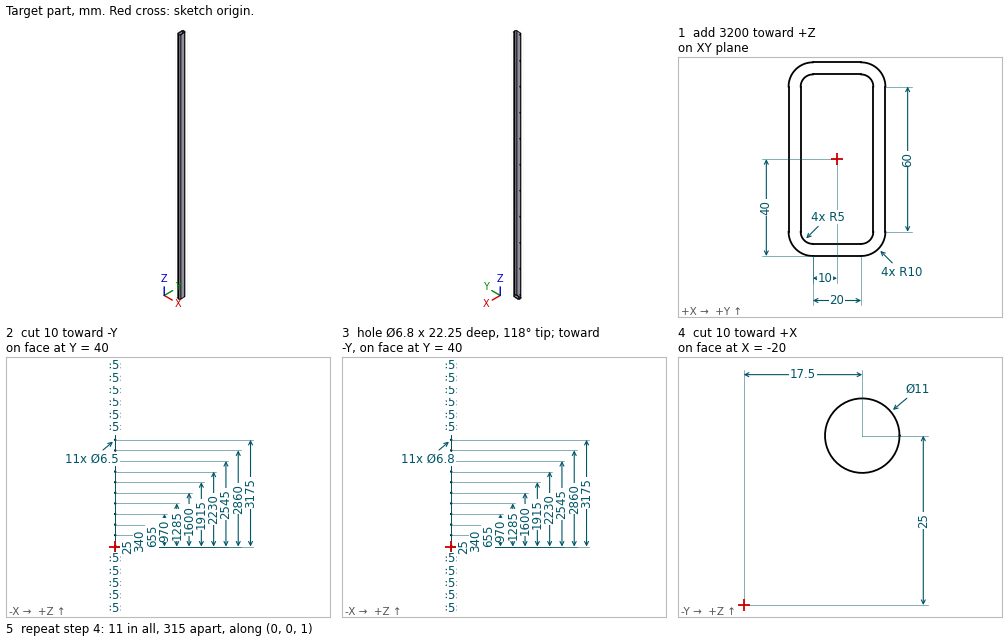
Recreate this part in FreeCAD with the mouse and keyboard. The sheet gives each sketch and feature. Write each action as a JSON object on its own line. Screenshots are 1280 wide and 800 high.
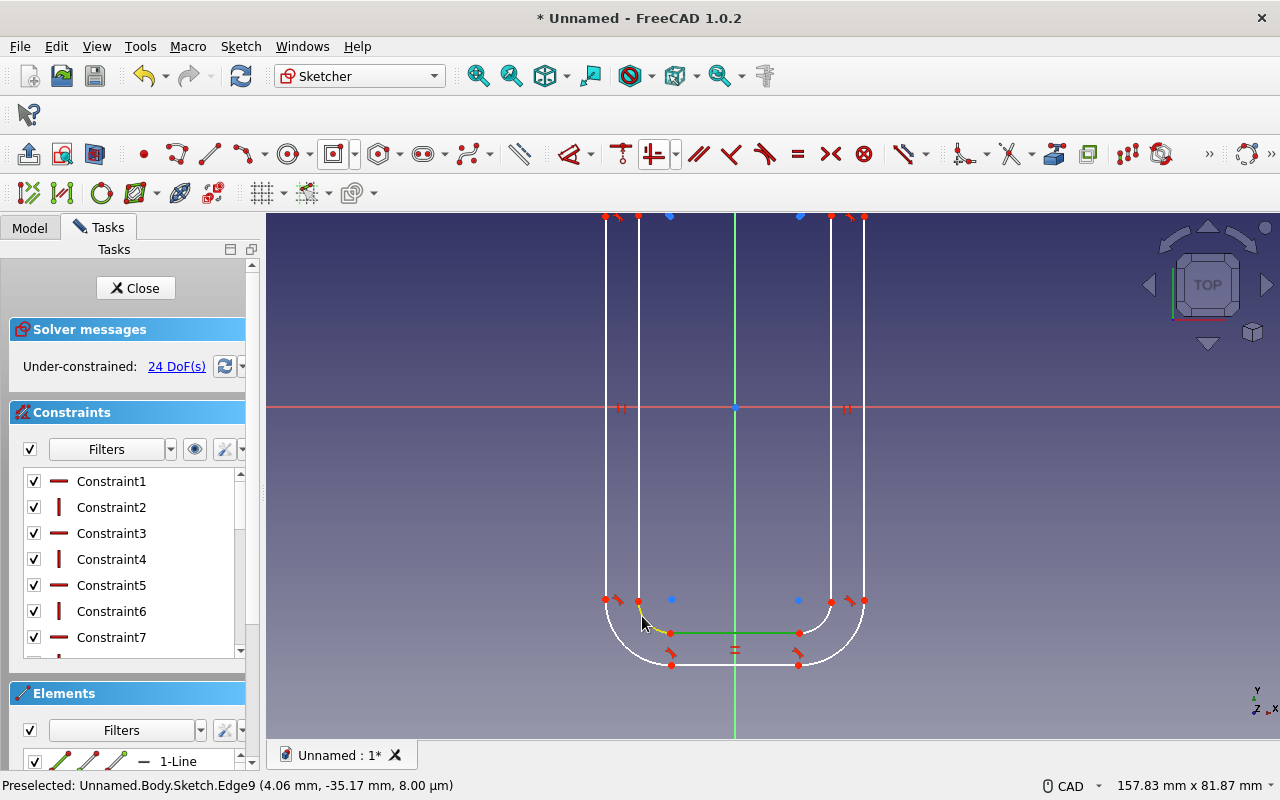
{"action": "left_click", "coordinate": [643, 616]}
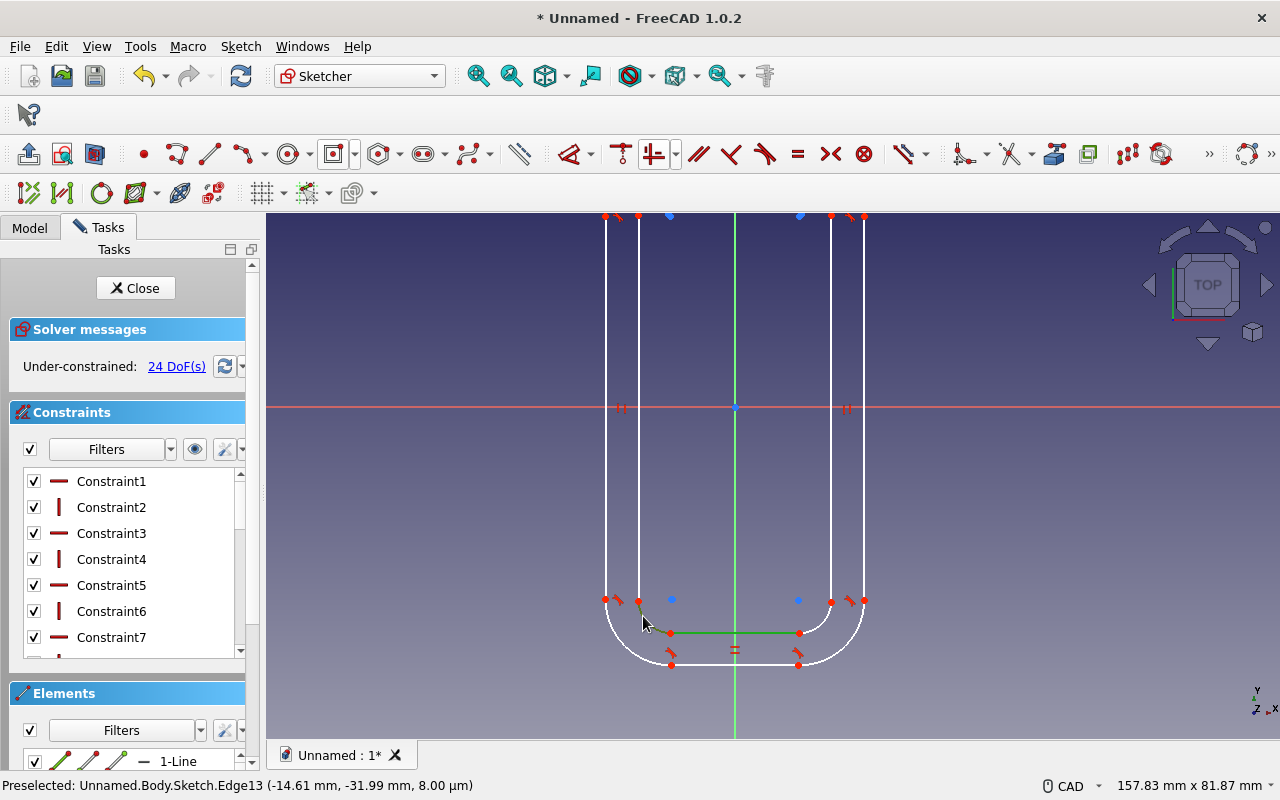
{"action": "left_click", "coordinate": [765, 154]}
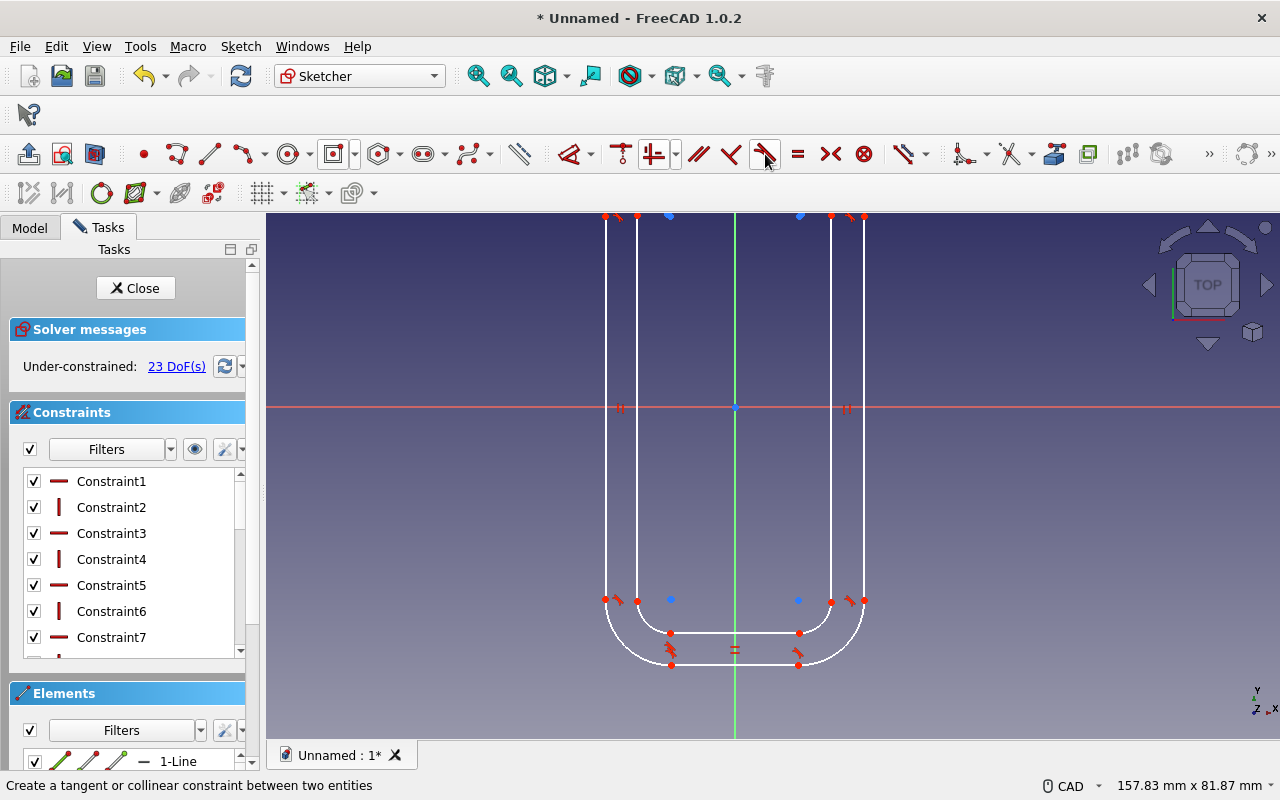
{"action": "left_click", "coordinate": [761, 633]}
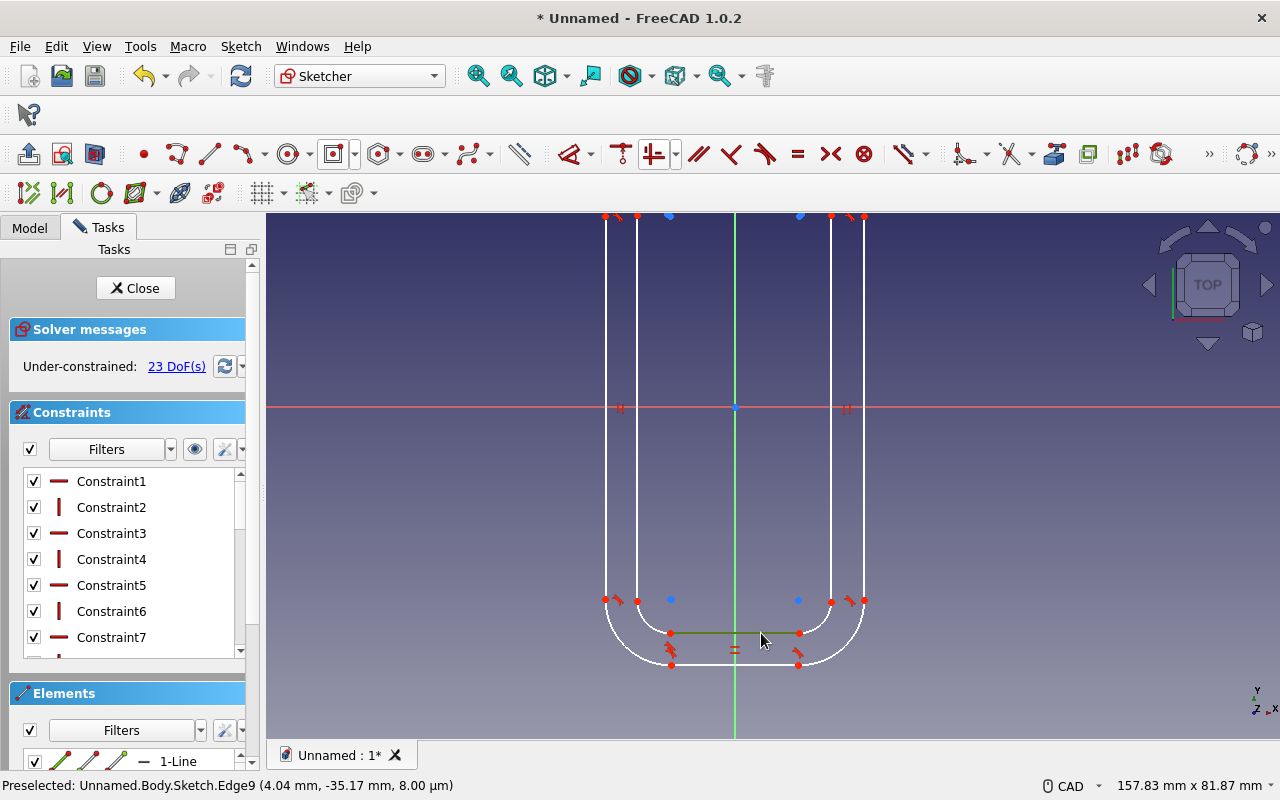
{"action": "left_click", "coordinate": [814, 630]}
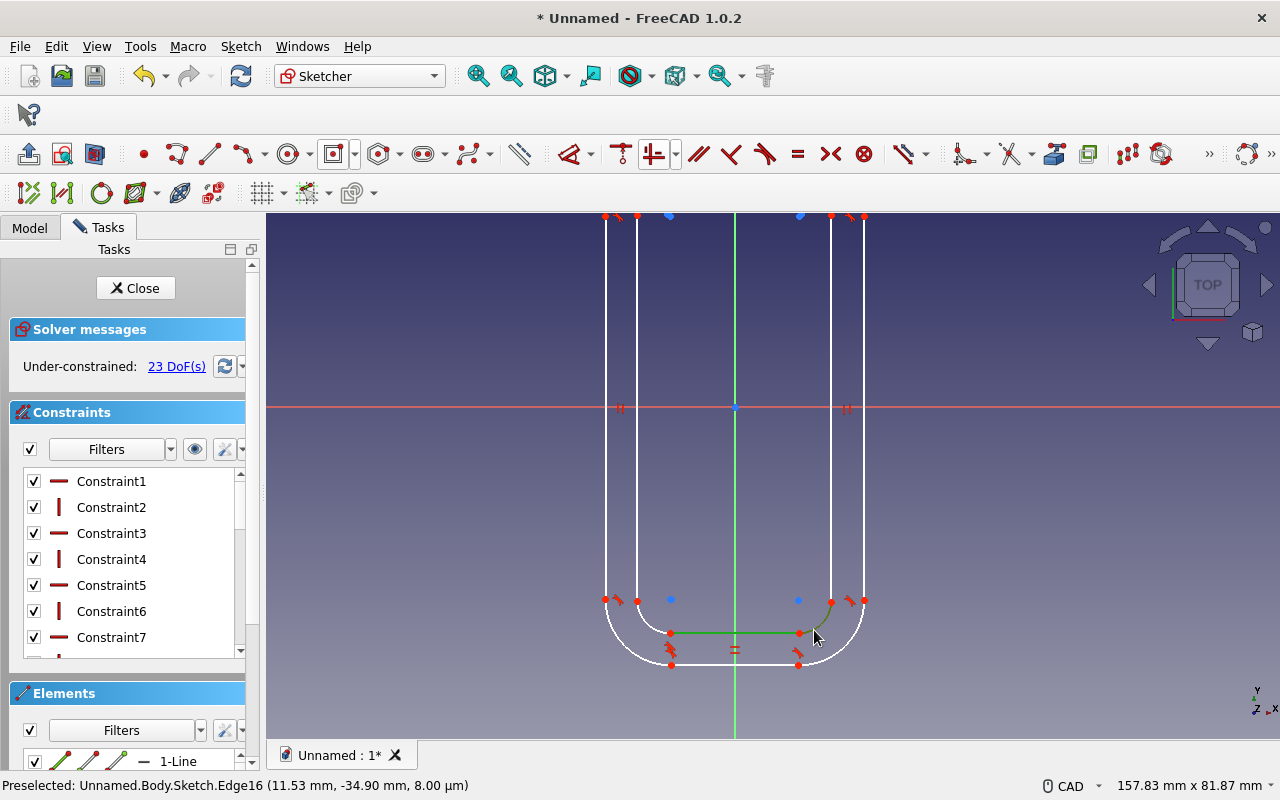
{"action": "left_click", "coordinate": [765, 154]}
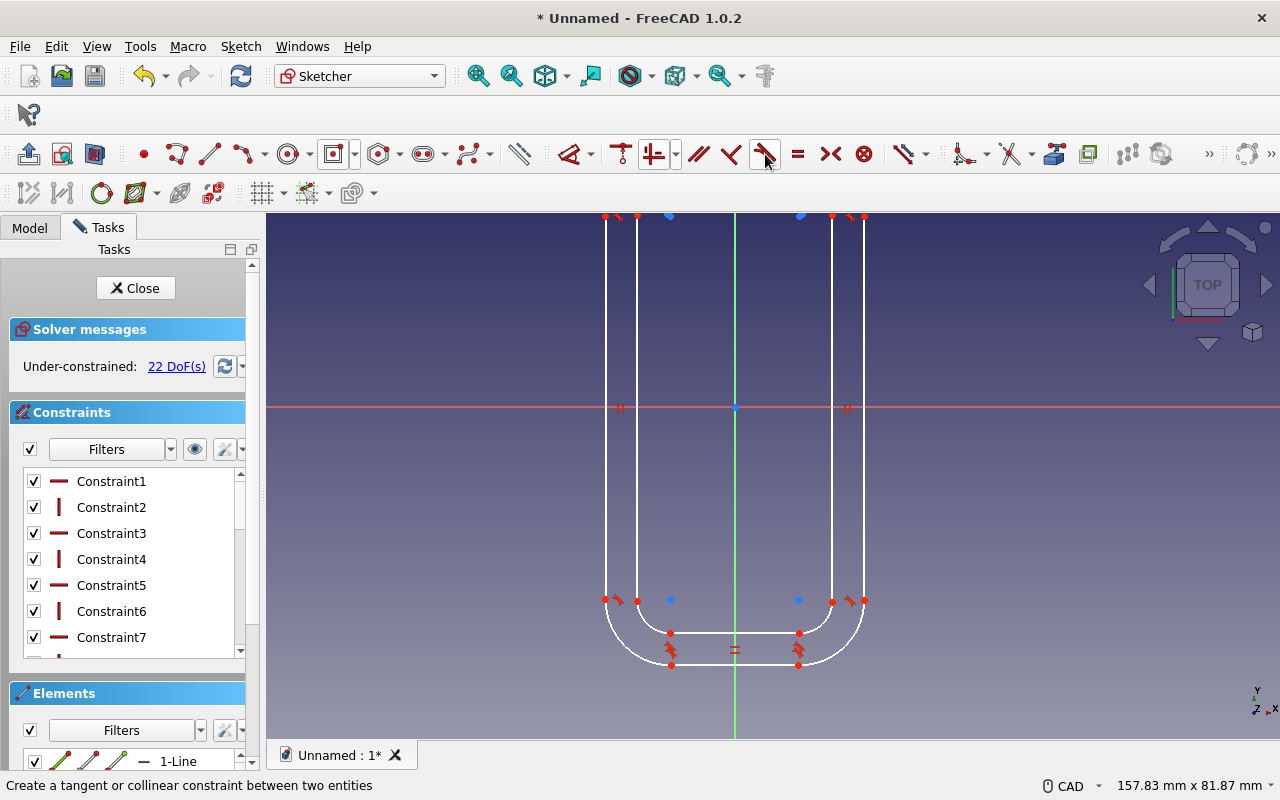
{"action": "left_click", "coordinate": [637, 486]}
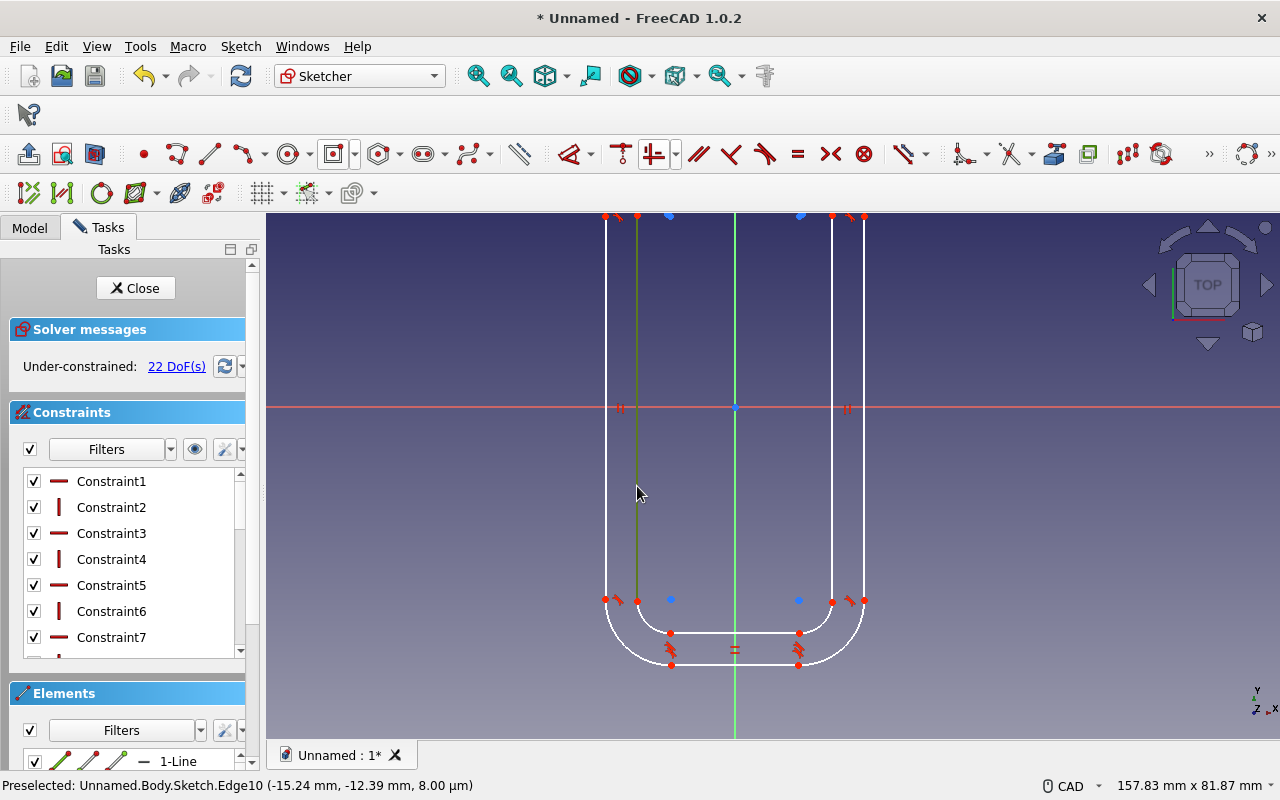
{"action": "left_click", "coordinate": [641, 616]}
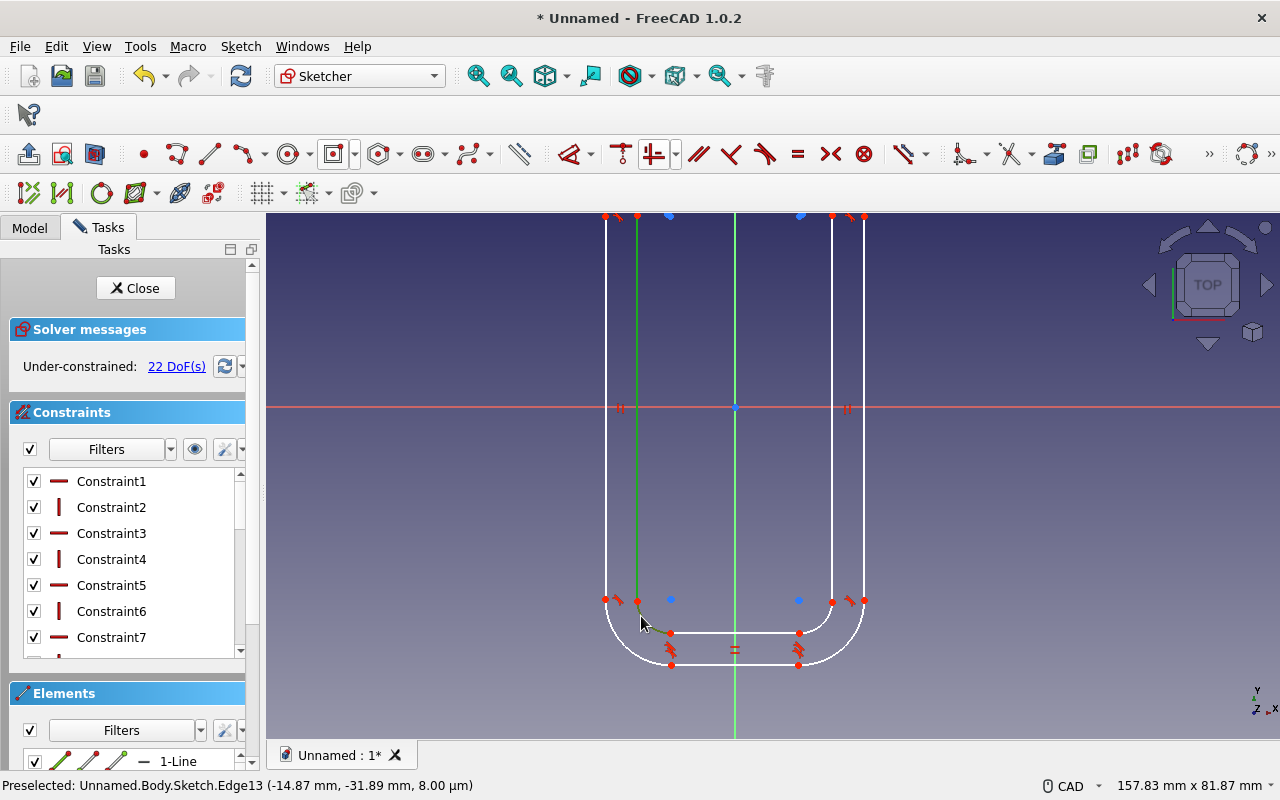
{"action": "left_click", "coordinate": [765, 154]}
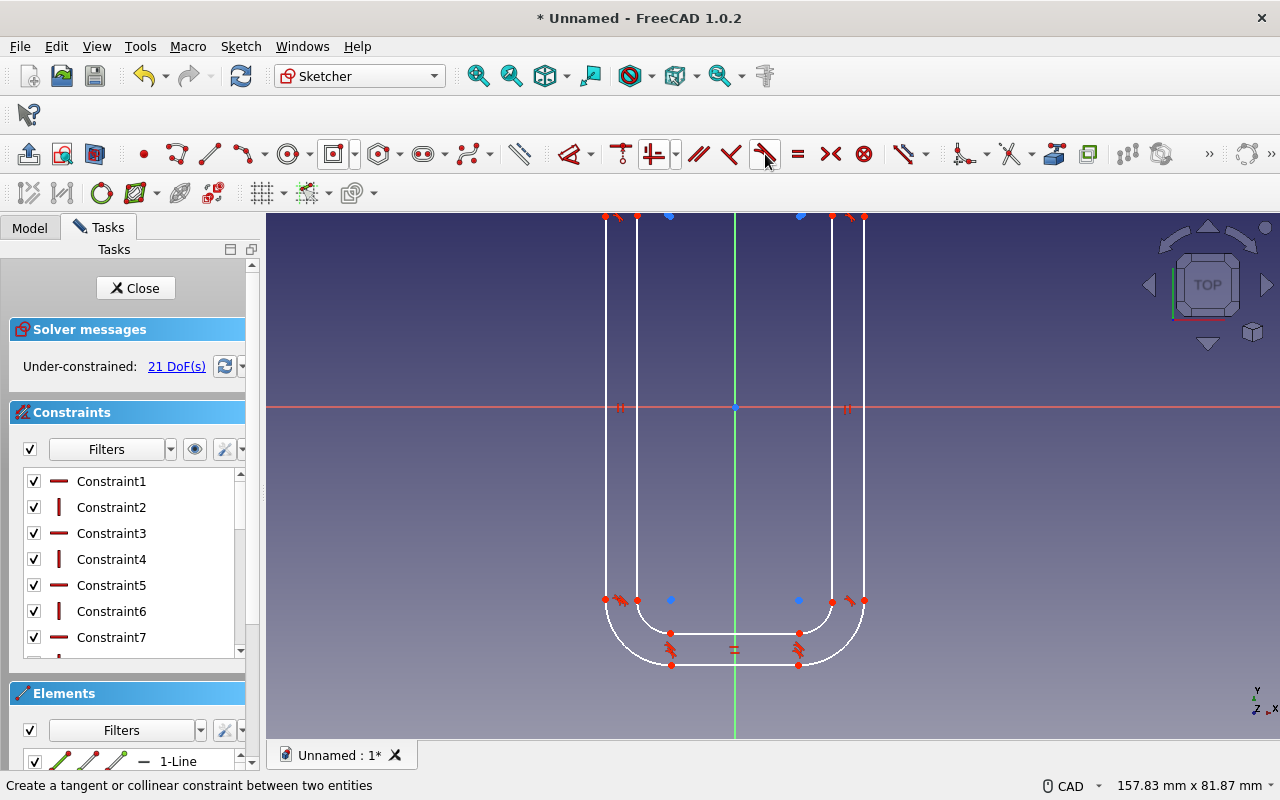
{"action": "left_click", "coordinate": [637, 485]}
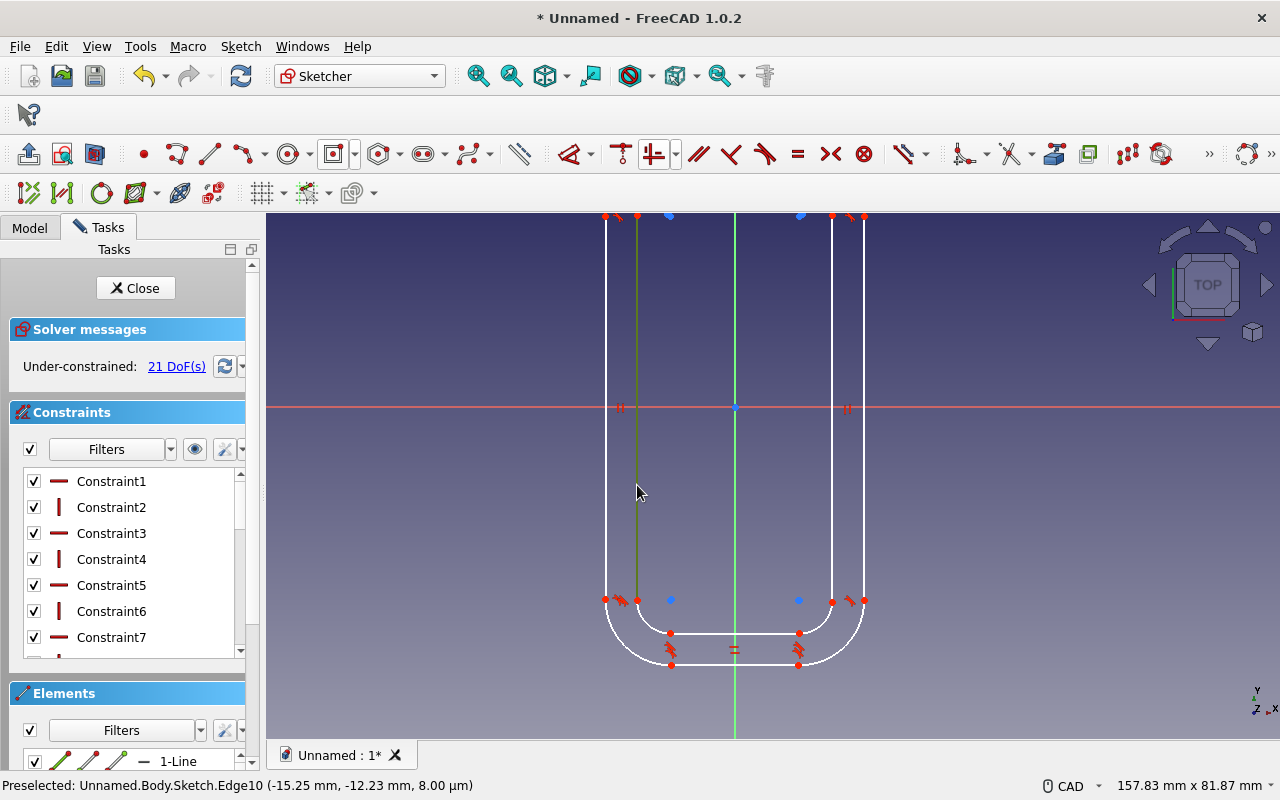
{"action": "scroll", "coordinate": [642, 615], "scroll_direction": "down", "scroll_amount": 2}